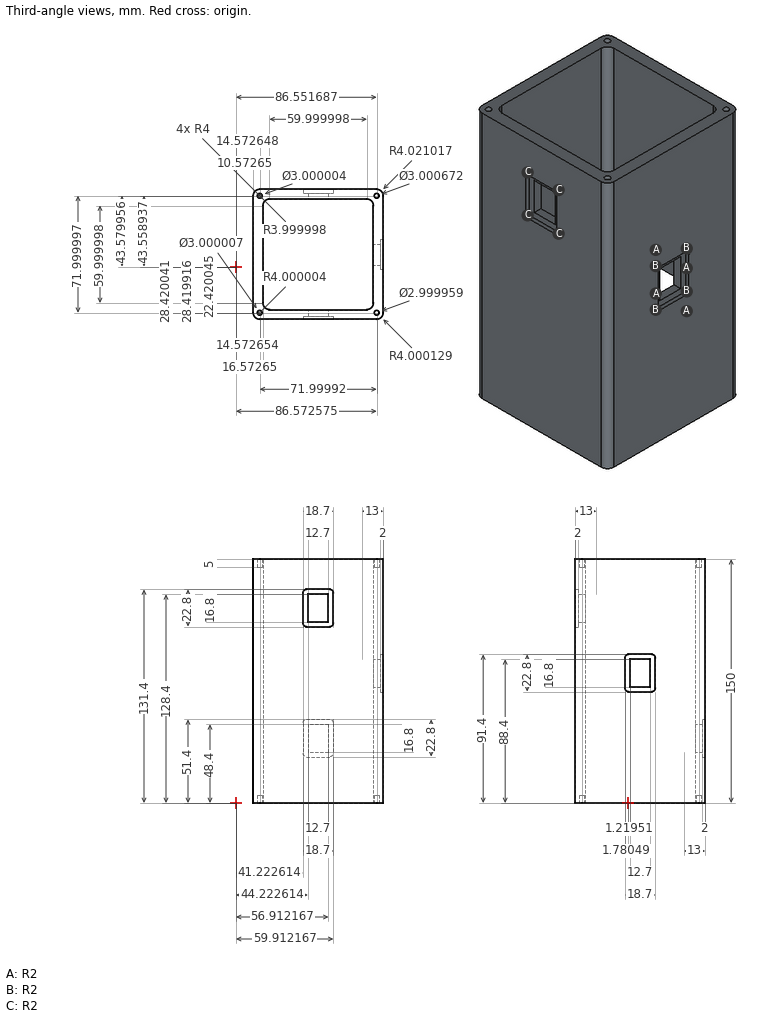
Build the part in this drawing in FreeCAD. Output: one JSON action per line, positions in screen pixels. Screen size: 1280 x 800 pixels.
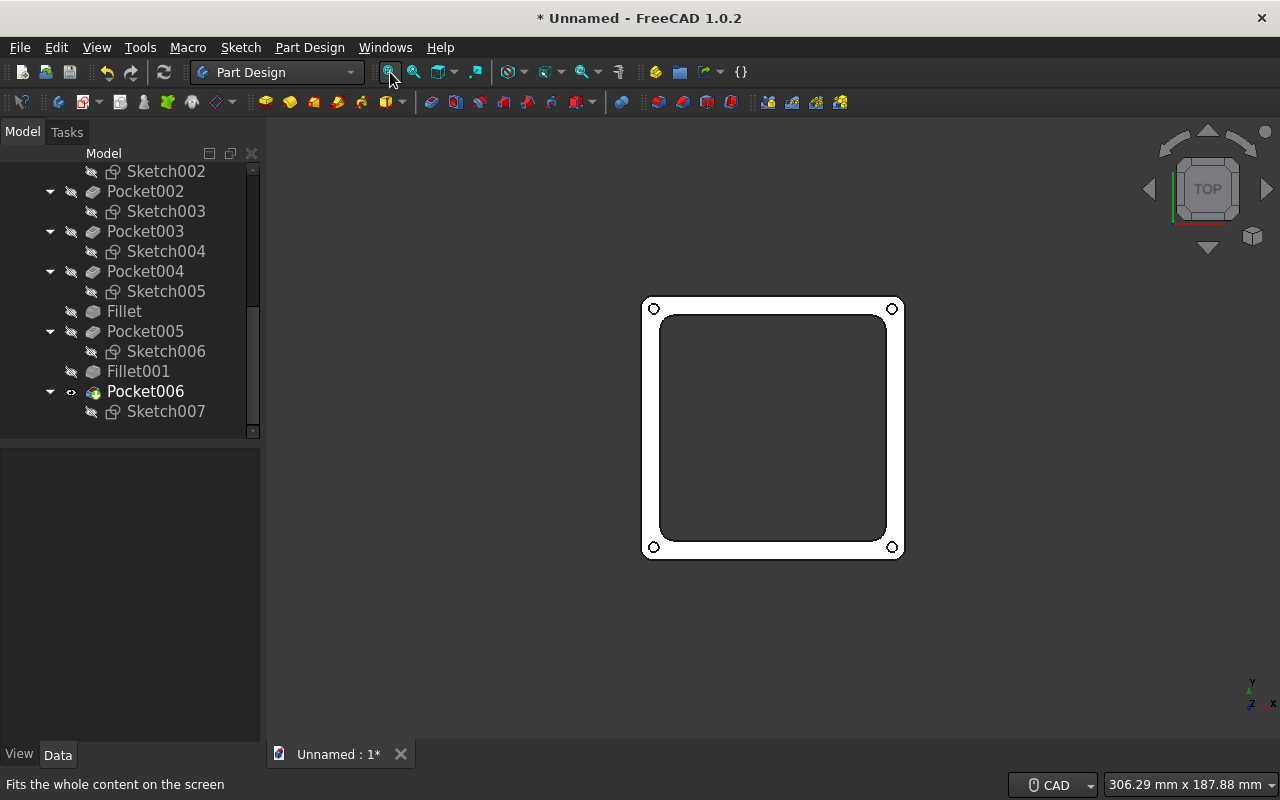
{"action": "scroll", "coordinate": [742, 556], "scroll_direction": "up", "scroll_amount": 9}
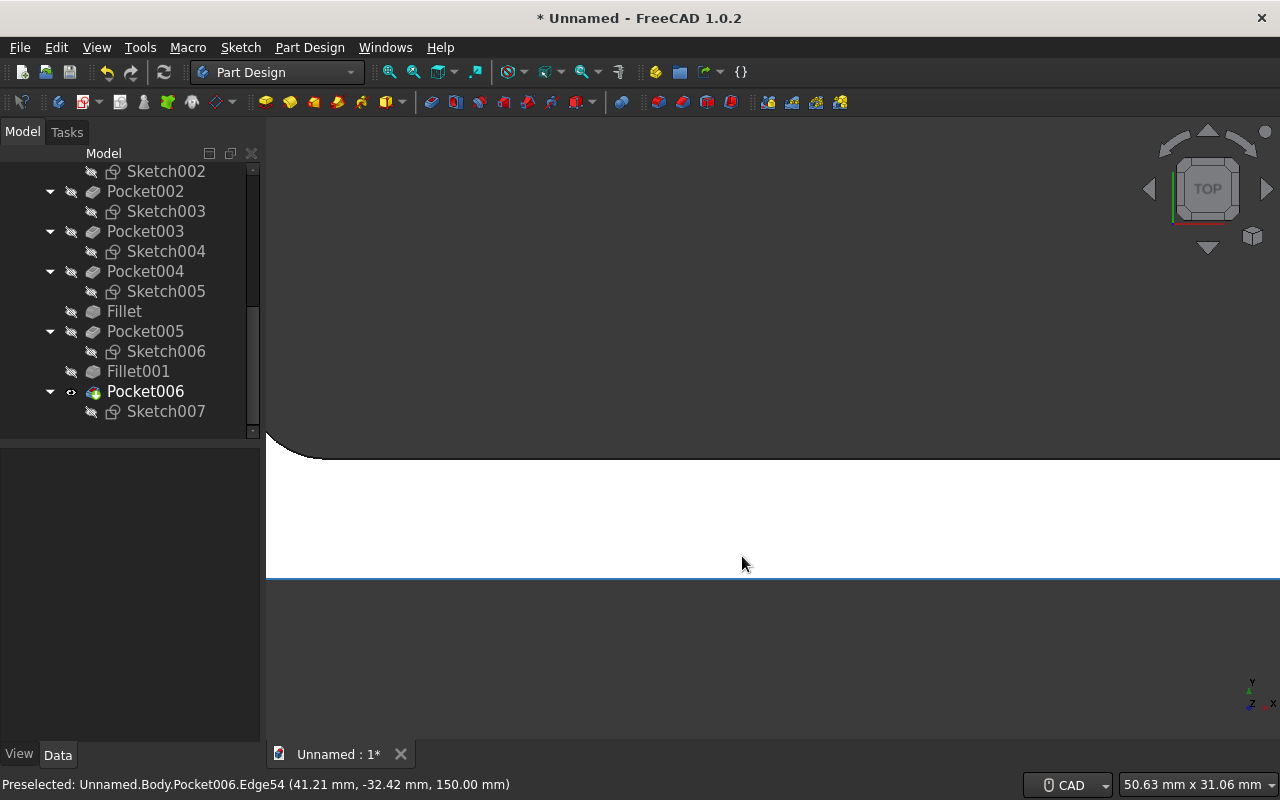
{"action": "left_click", "coordinate": [390, 72]}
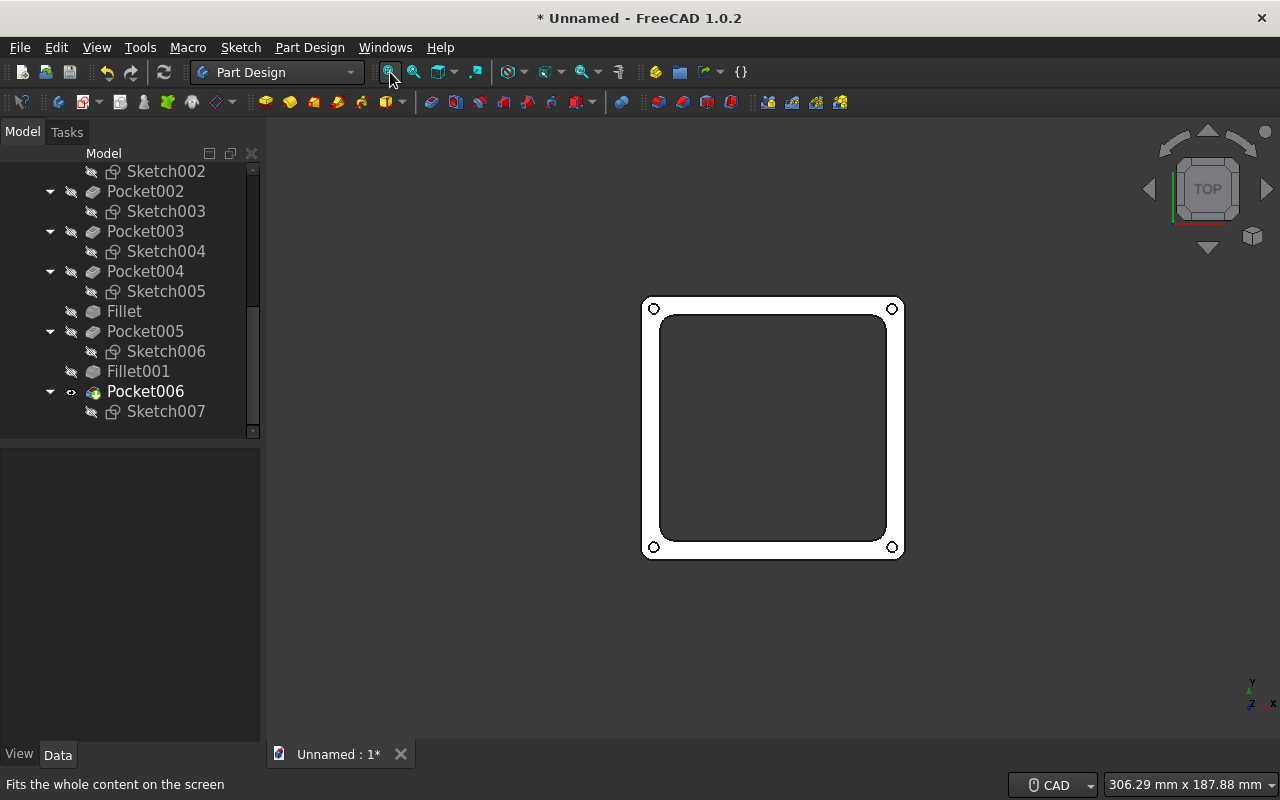
{"action": "key", "text": "0"}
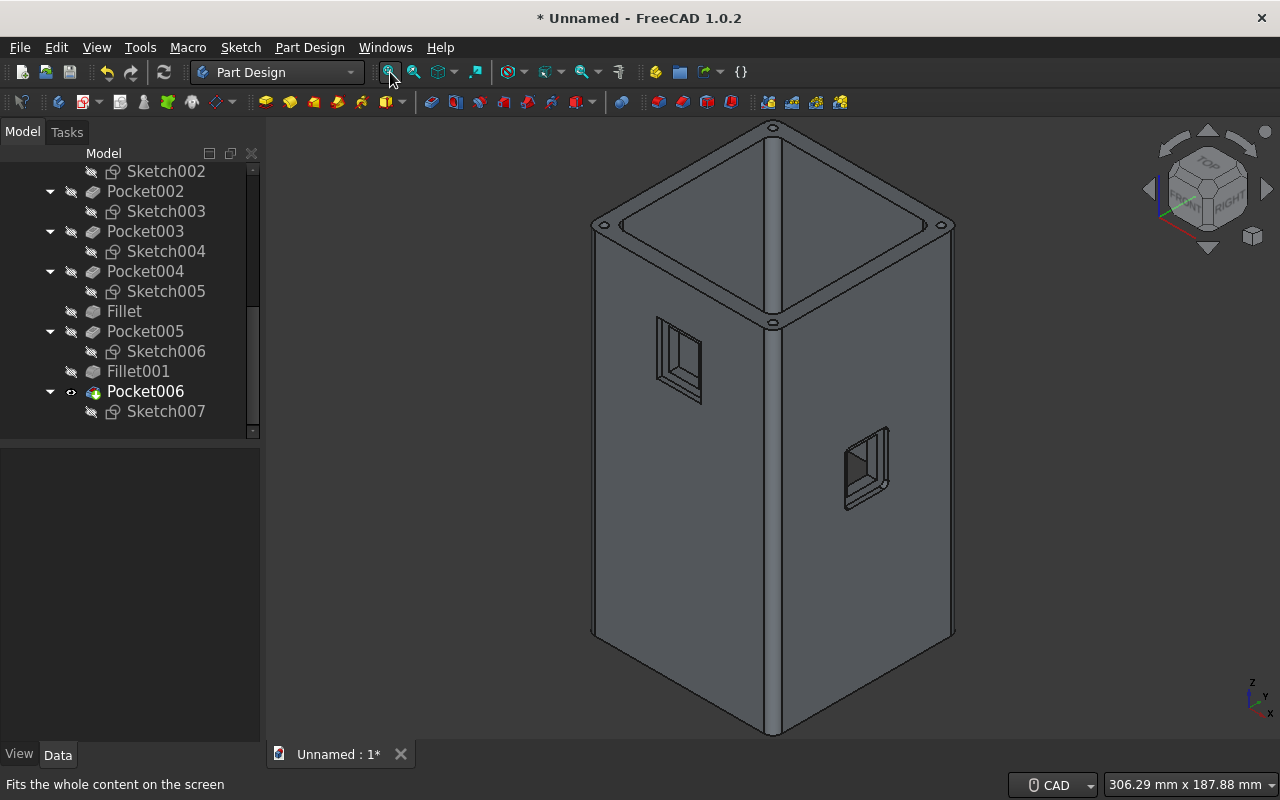
{"action": "left_click", "coordinate": [390, 72]}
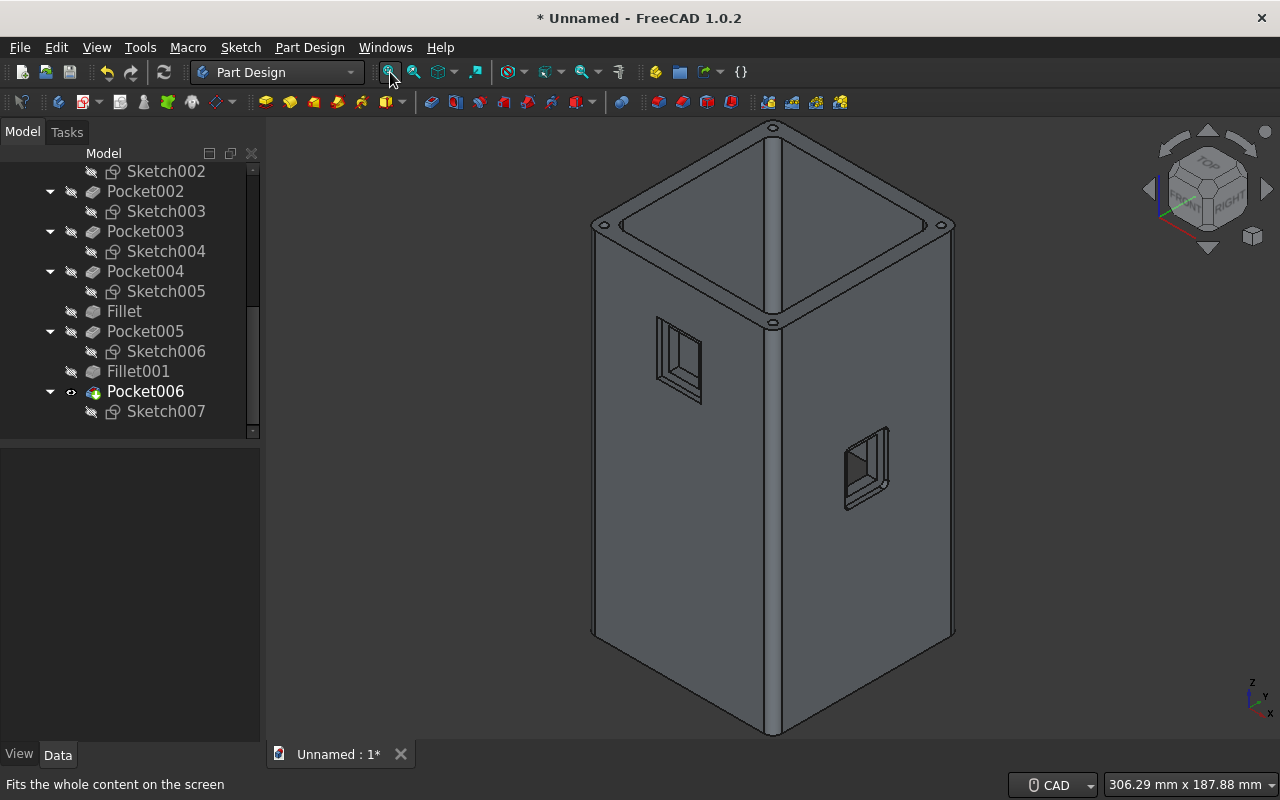
{"action": "scroll", "coordinate": [660, 376], "scroll_direction": "up", "scroll_amount": 9}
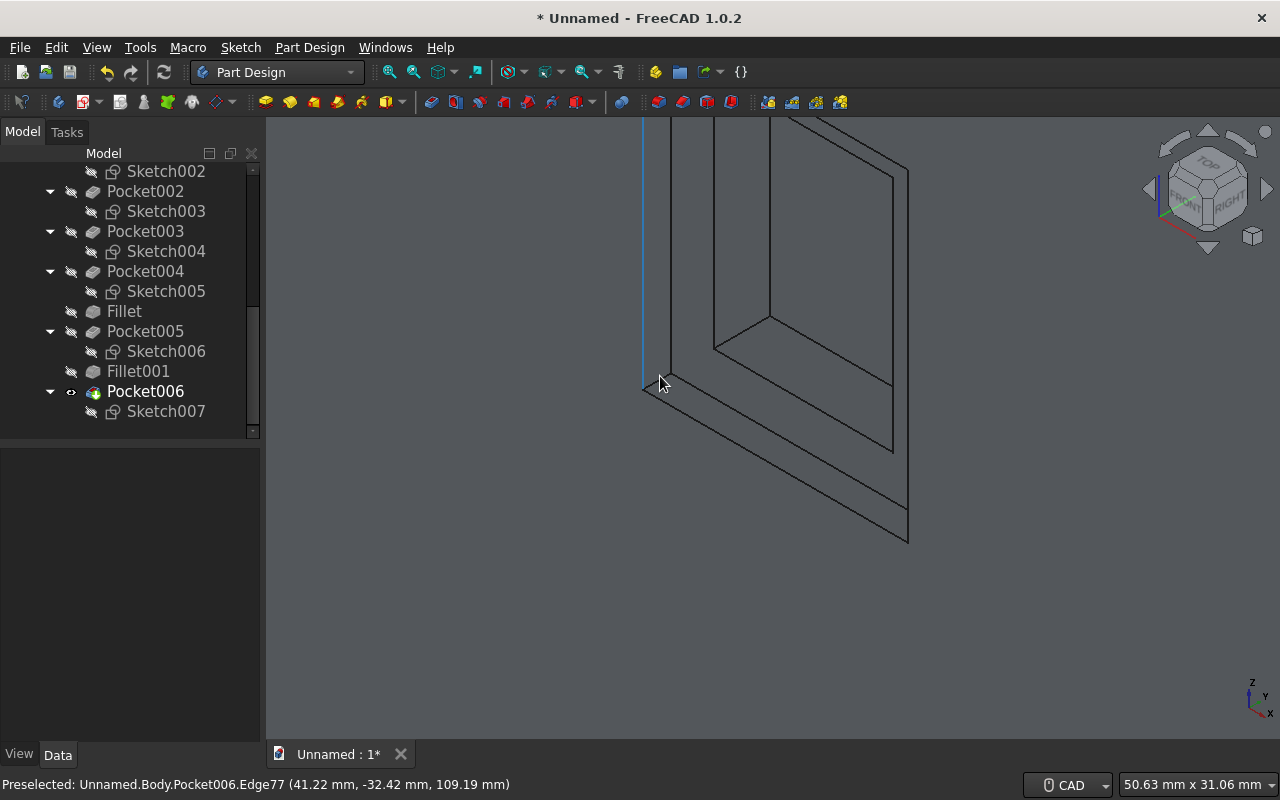
{"action": "key", "text": "v f"}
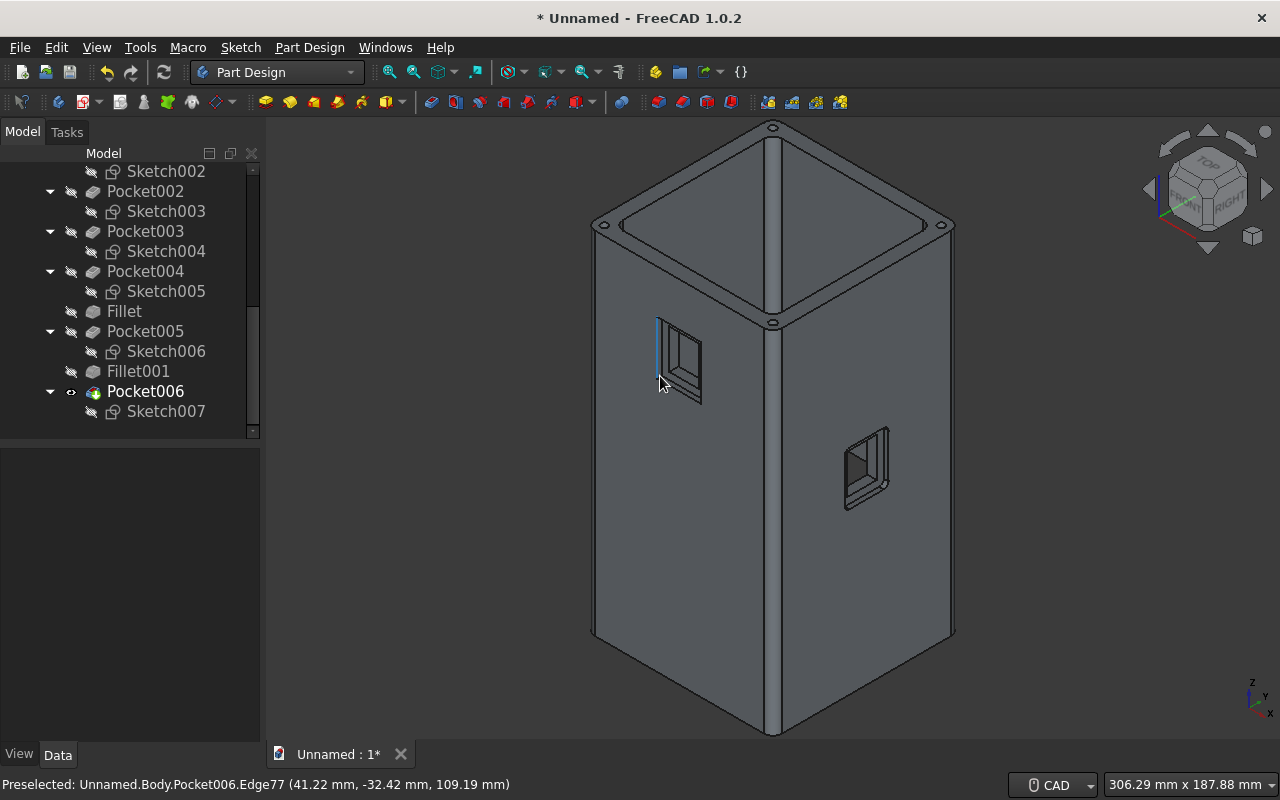
{"action": "key", "text": "1"}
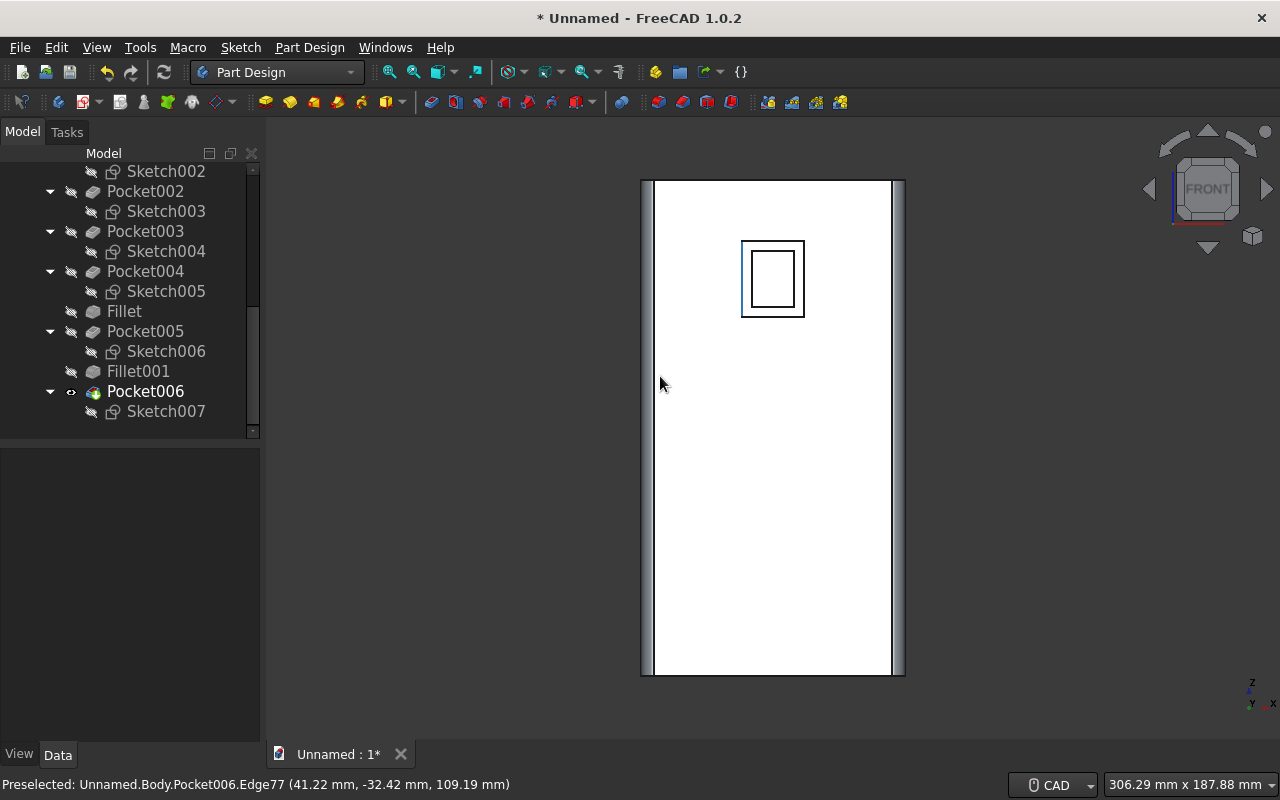
{"action": "scroll", "coordinate": [742, 316], "scroll_direction": "up", "scroll_amount": 9}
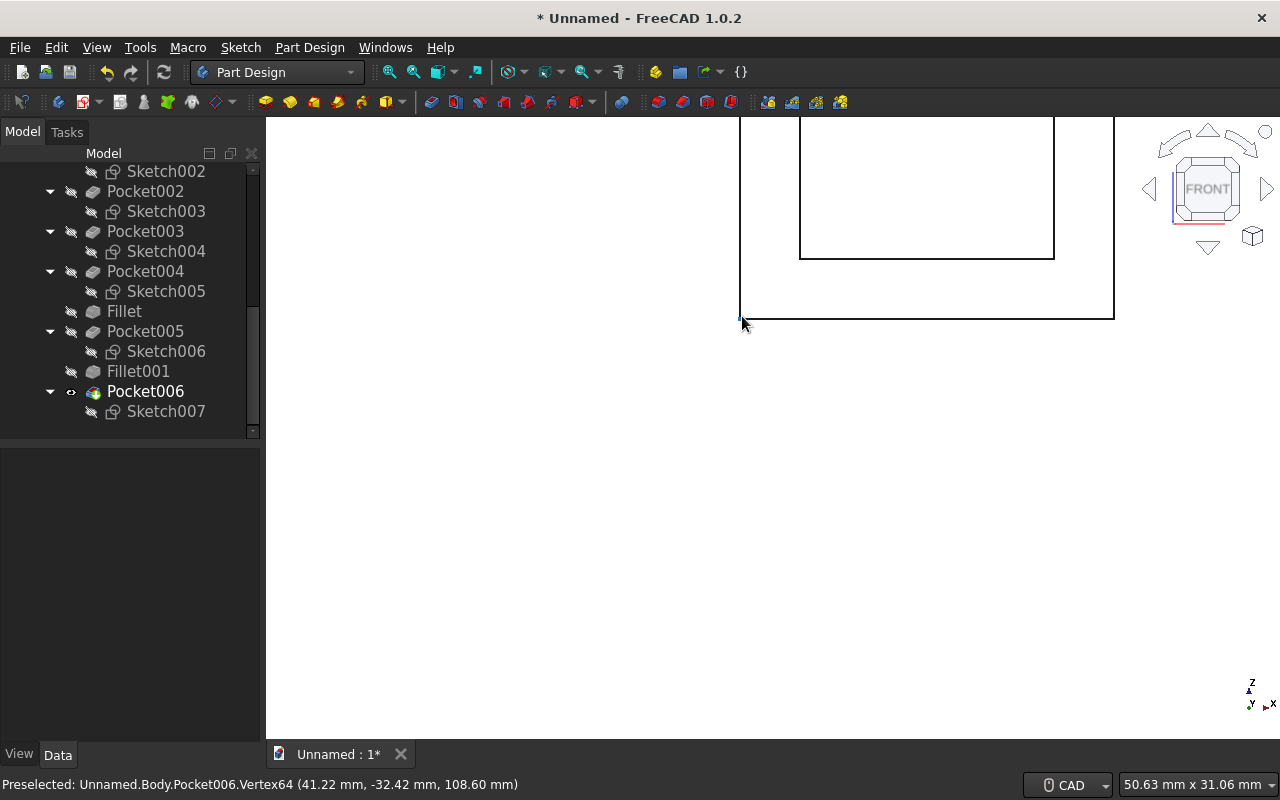
{"action": "left_click", "coordinate": [390, 72]}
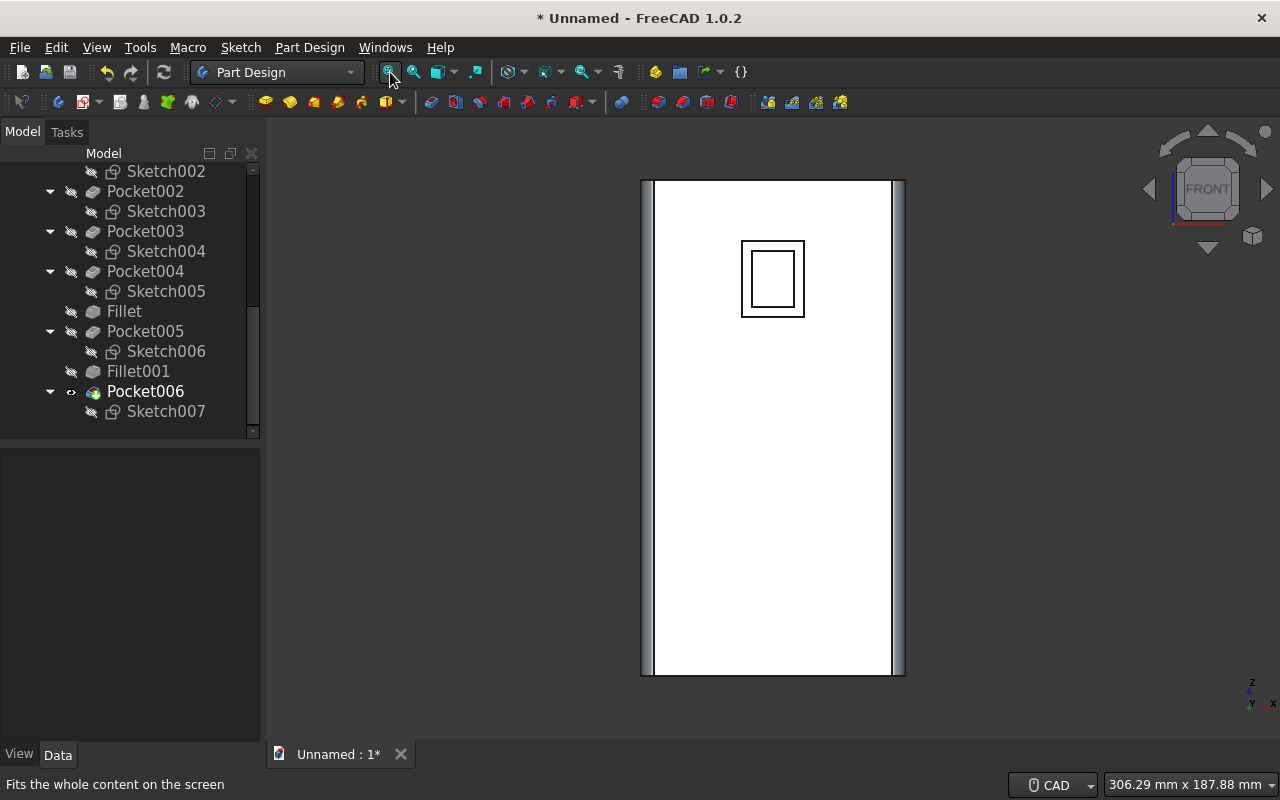
{"action": "key", "text": "3"}